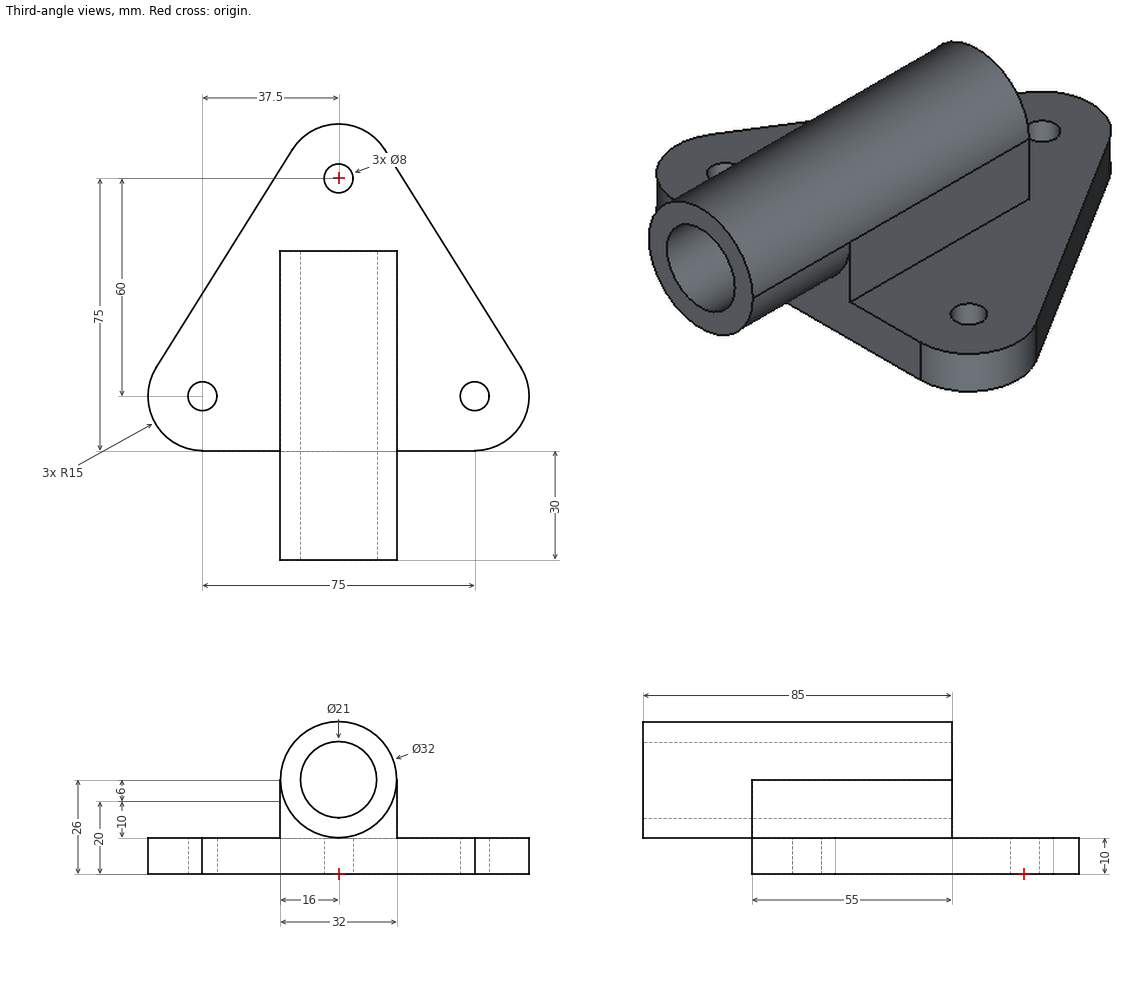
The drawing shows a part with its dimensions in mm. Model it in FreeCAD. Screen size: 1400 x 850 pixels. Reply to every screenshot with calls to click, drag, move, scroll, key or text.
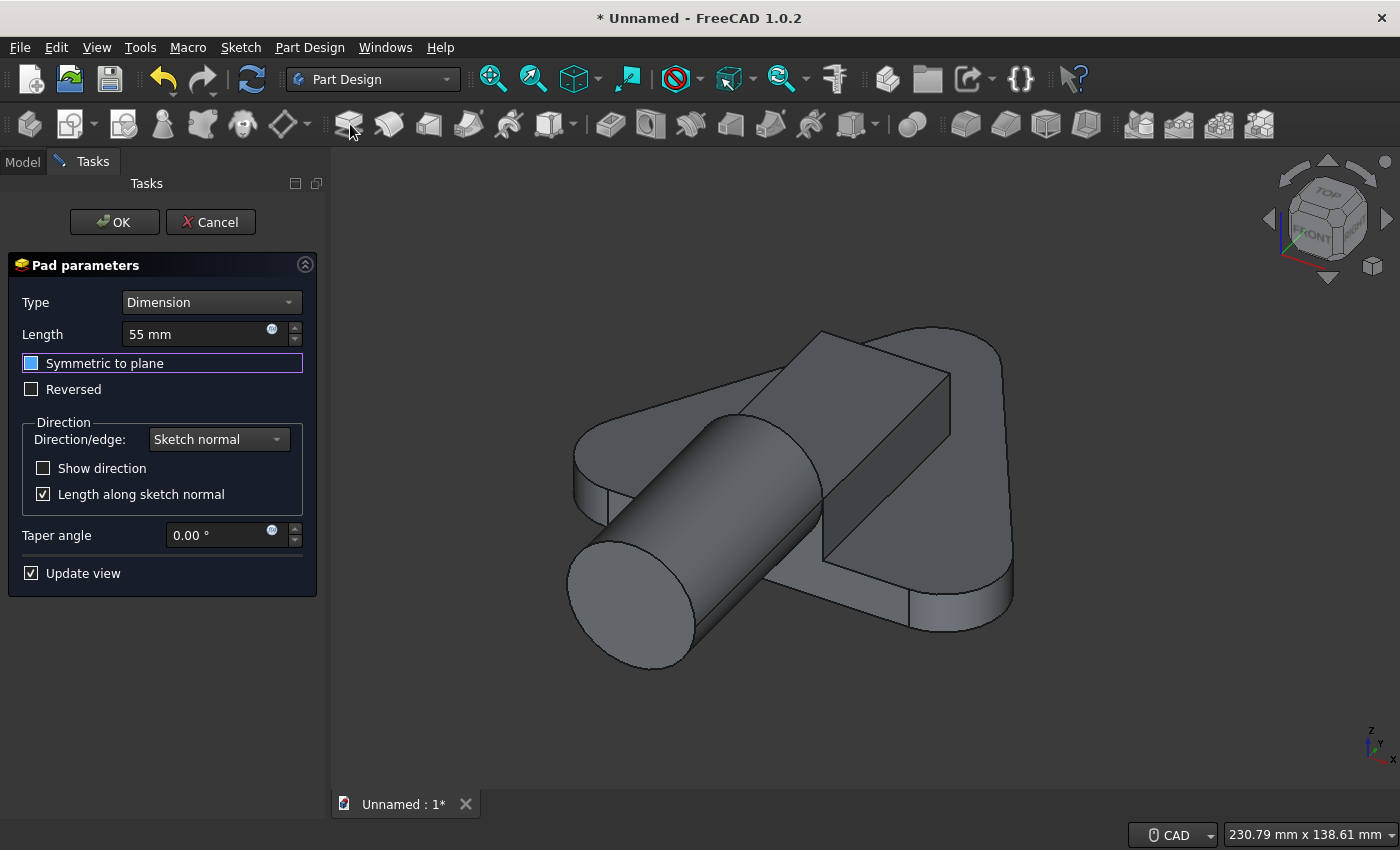
click(30, 389)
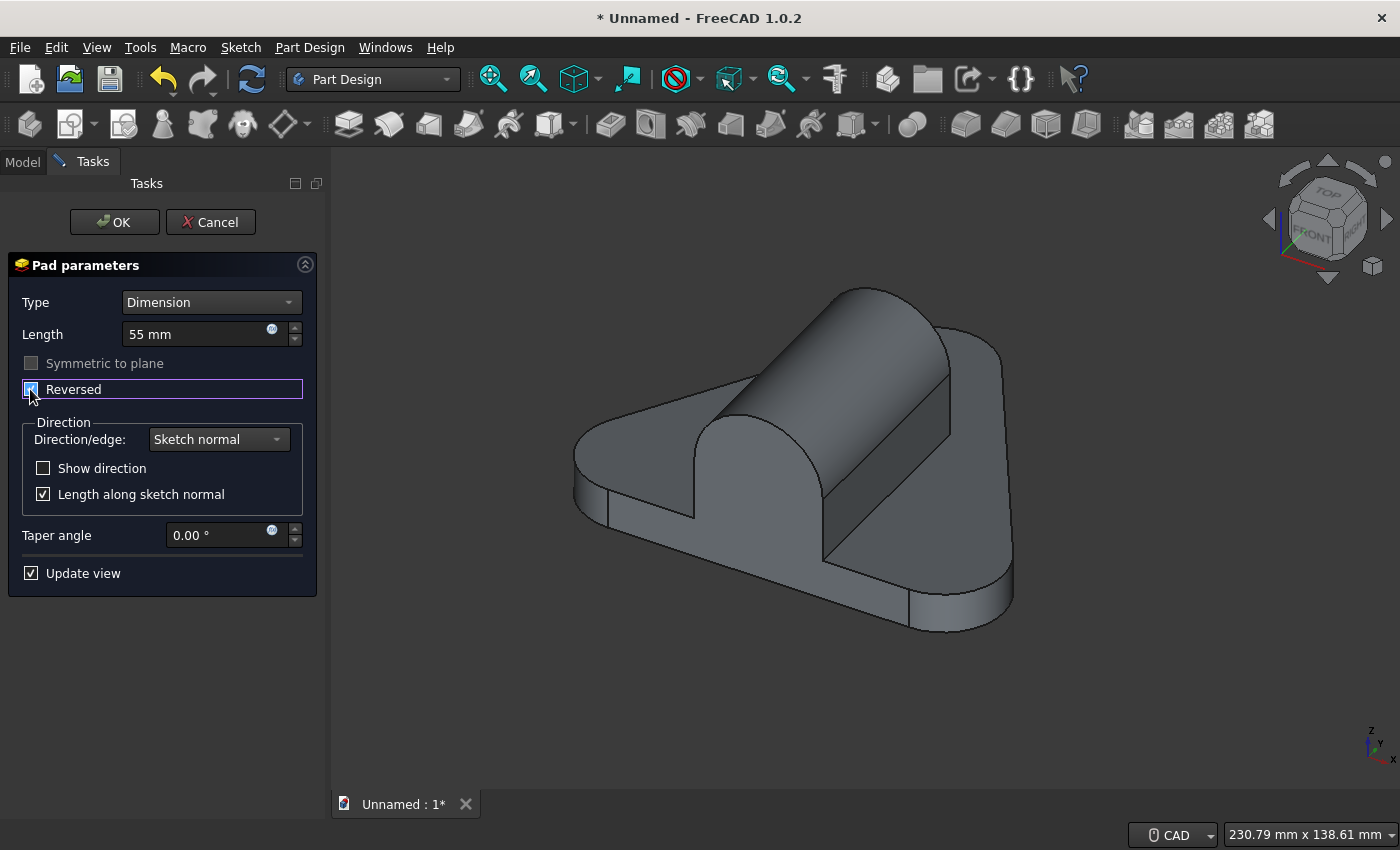
click(115, 222)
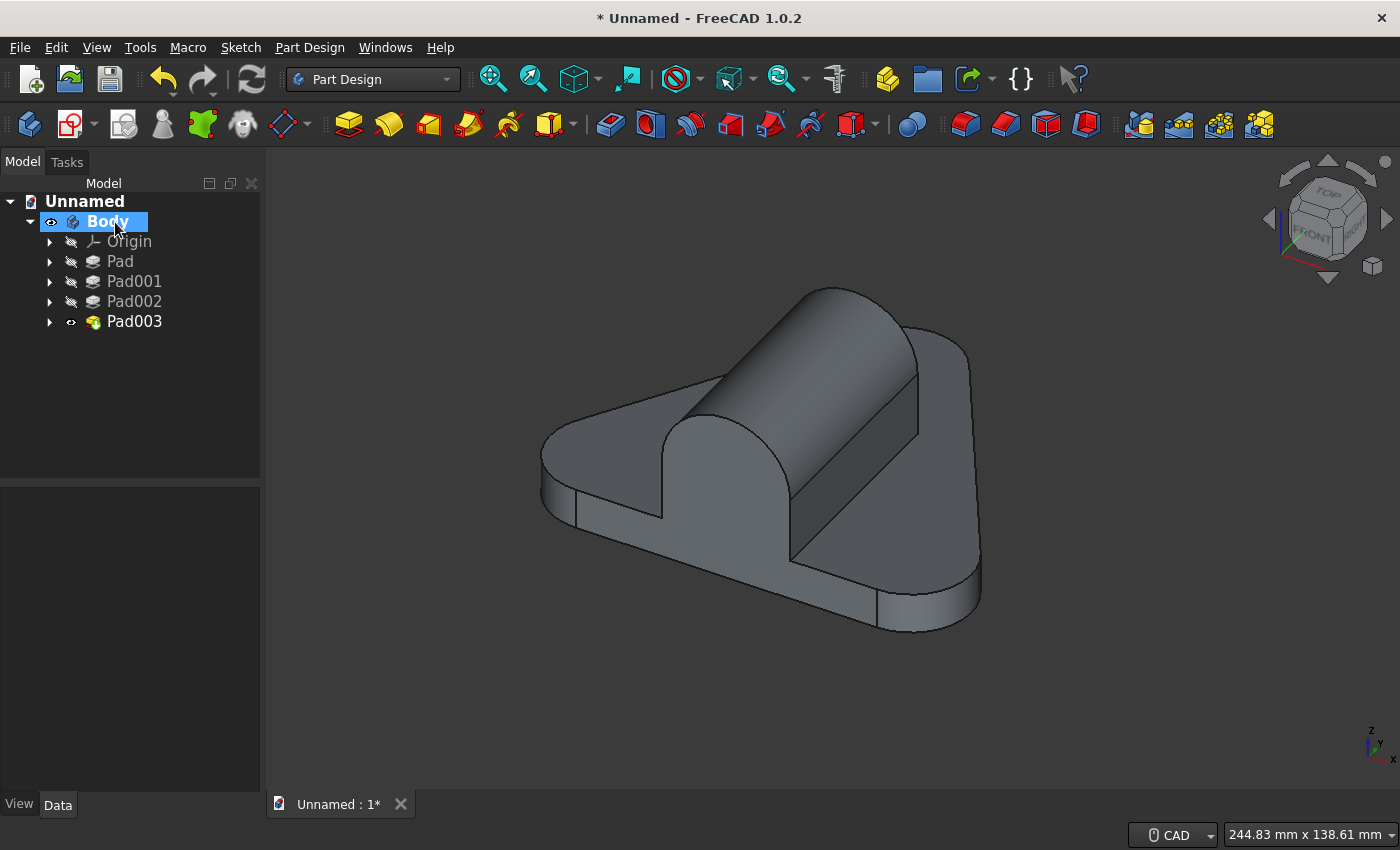
click(494, 80)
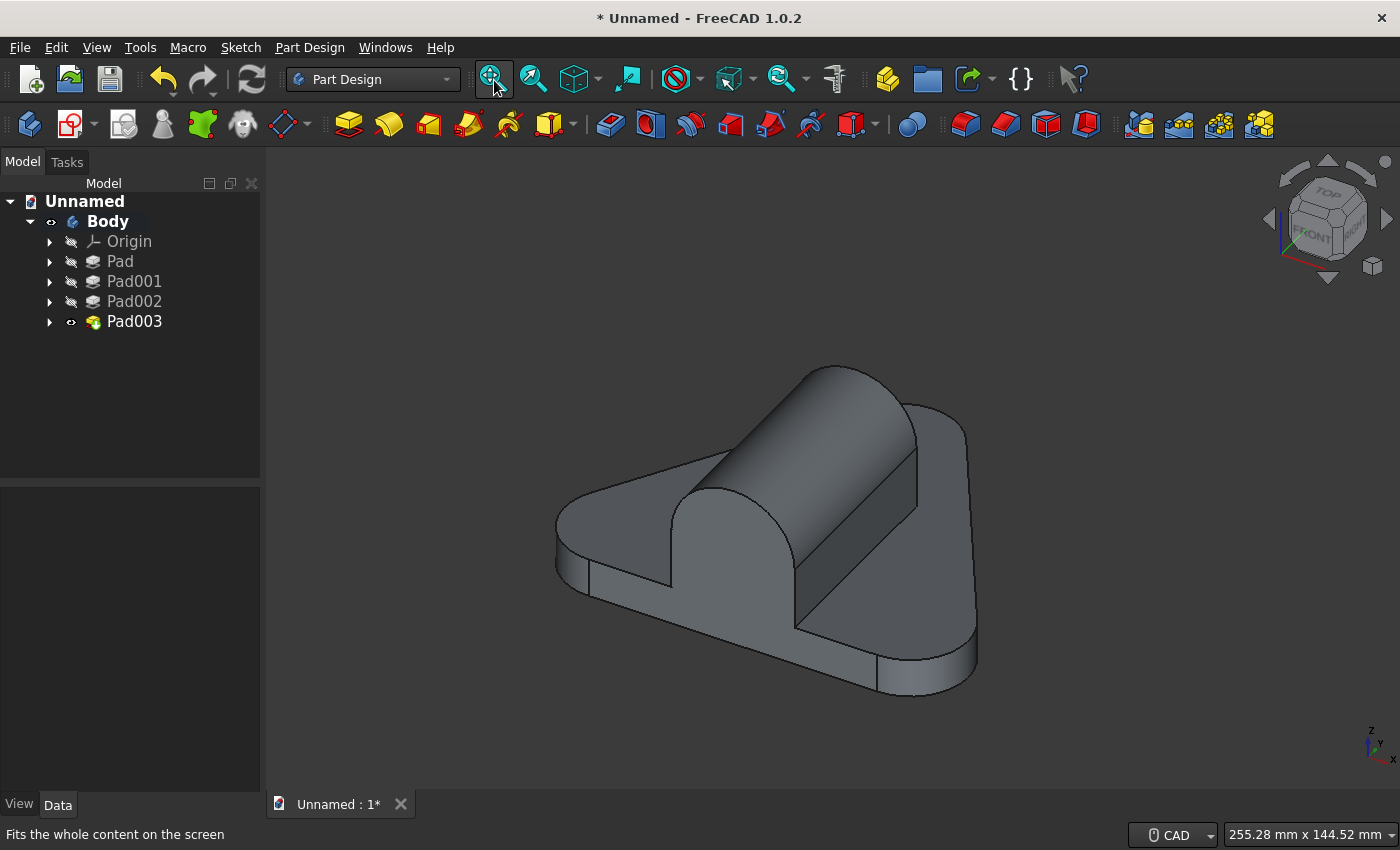
click(50, 242)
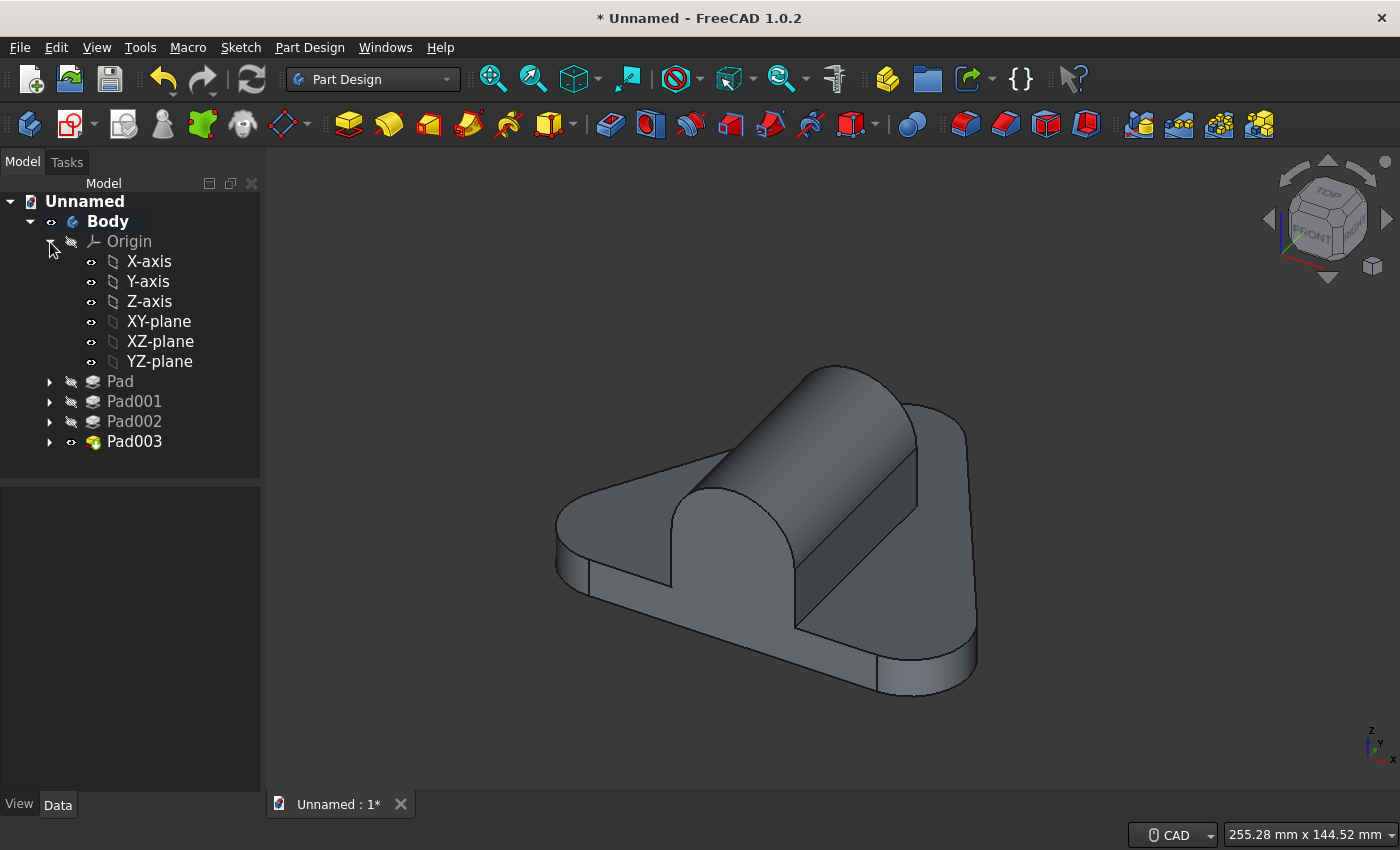
click(136, 342)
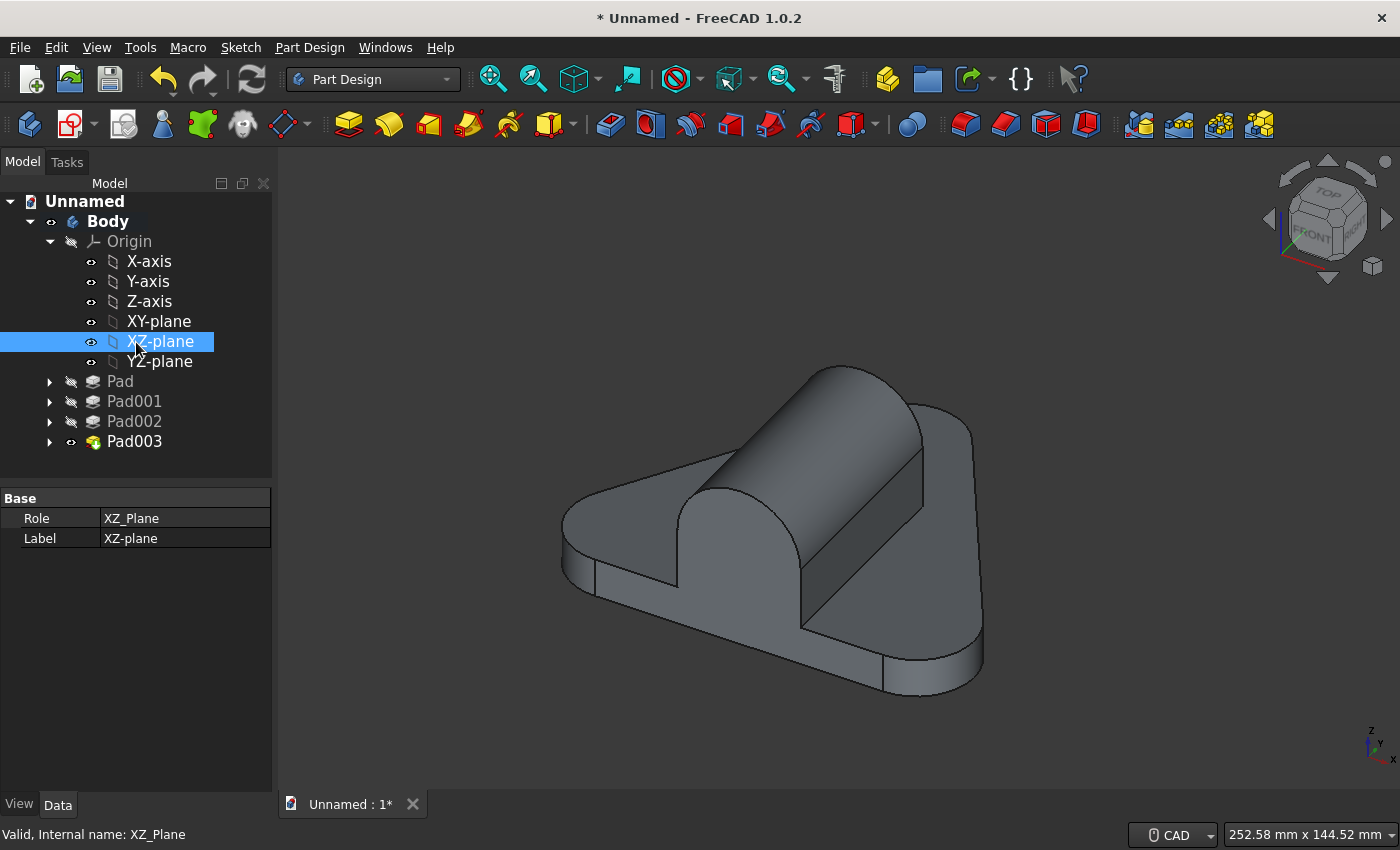
click(284, 124)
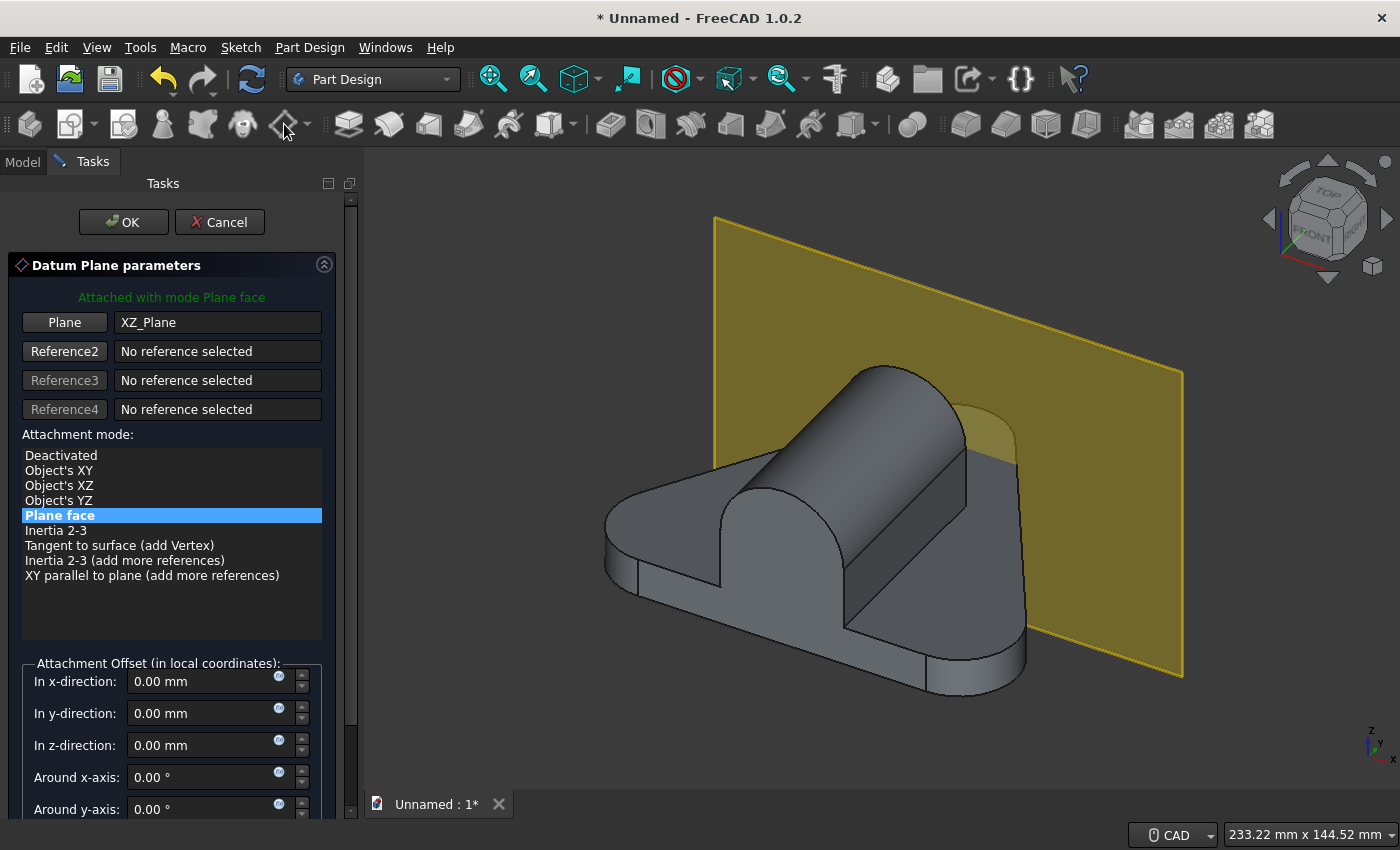
triple_click(210, 745)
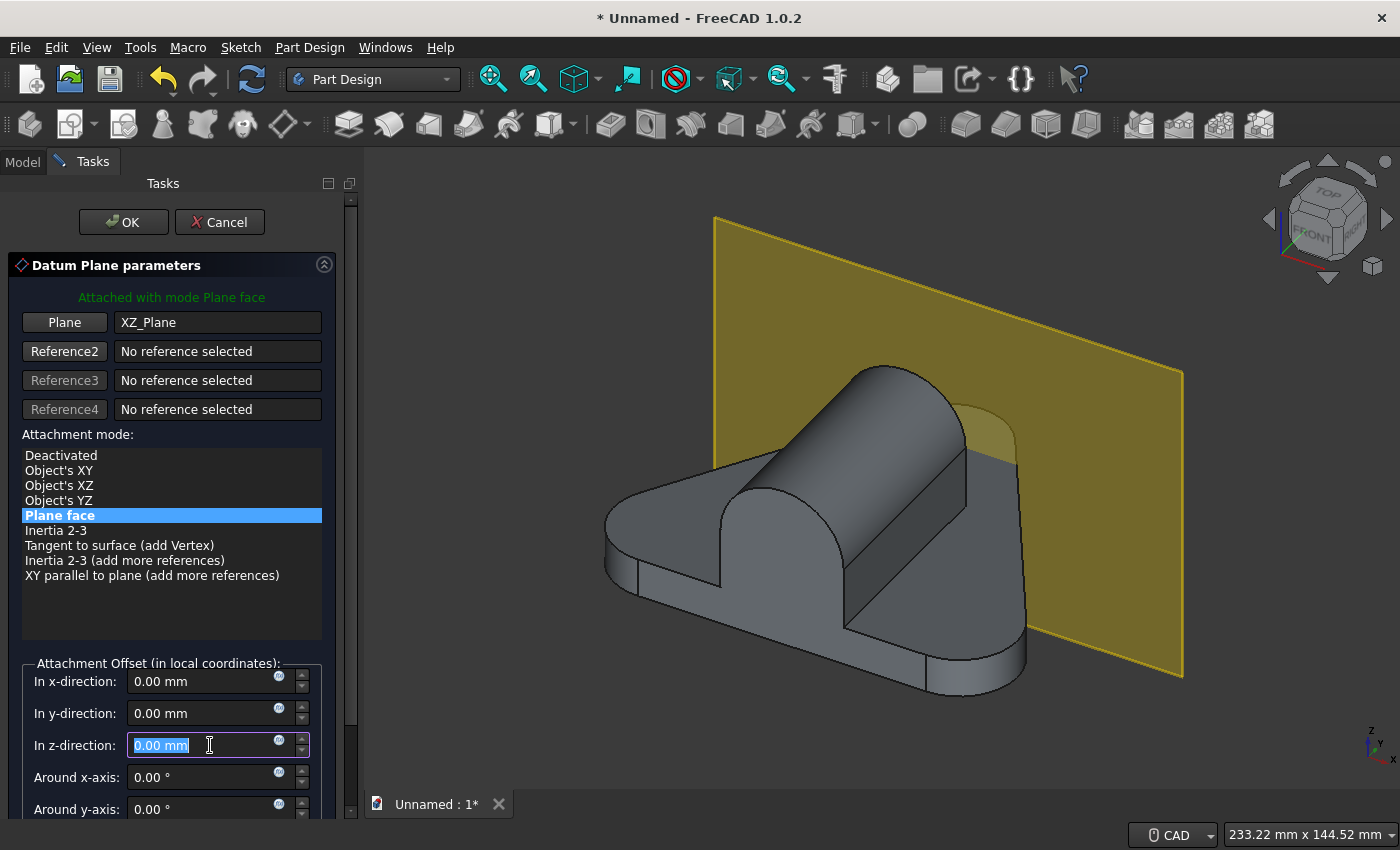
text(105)
key(Tab)